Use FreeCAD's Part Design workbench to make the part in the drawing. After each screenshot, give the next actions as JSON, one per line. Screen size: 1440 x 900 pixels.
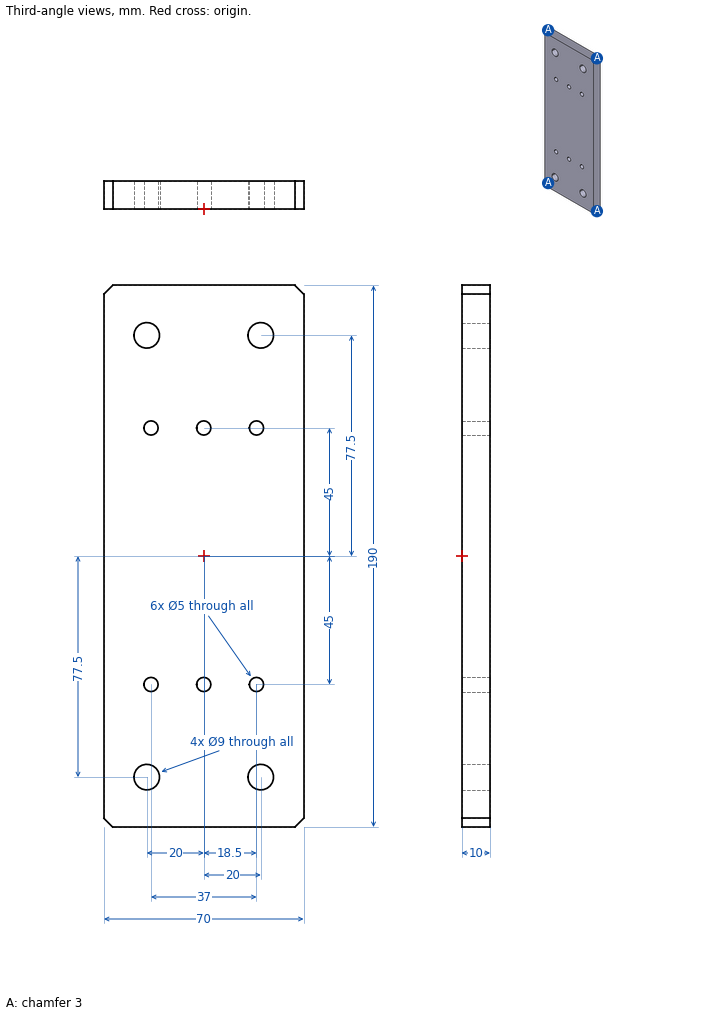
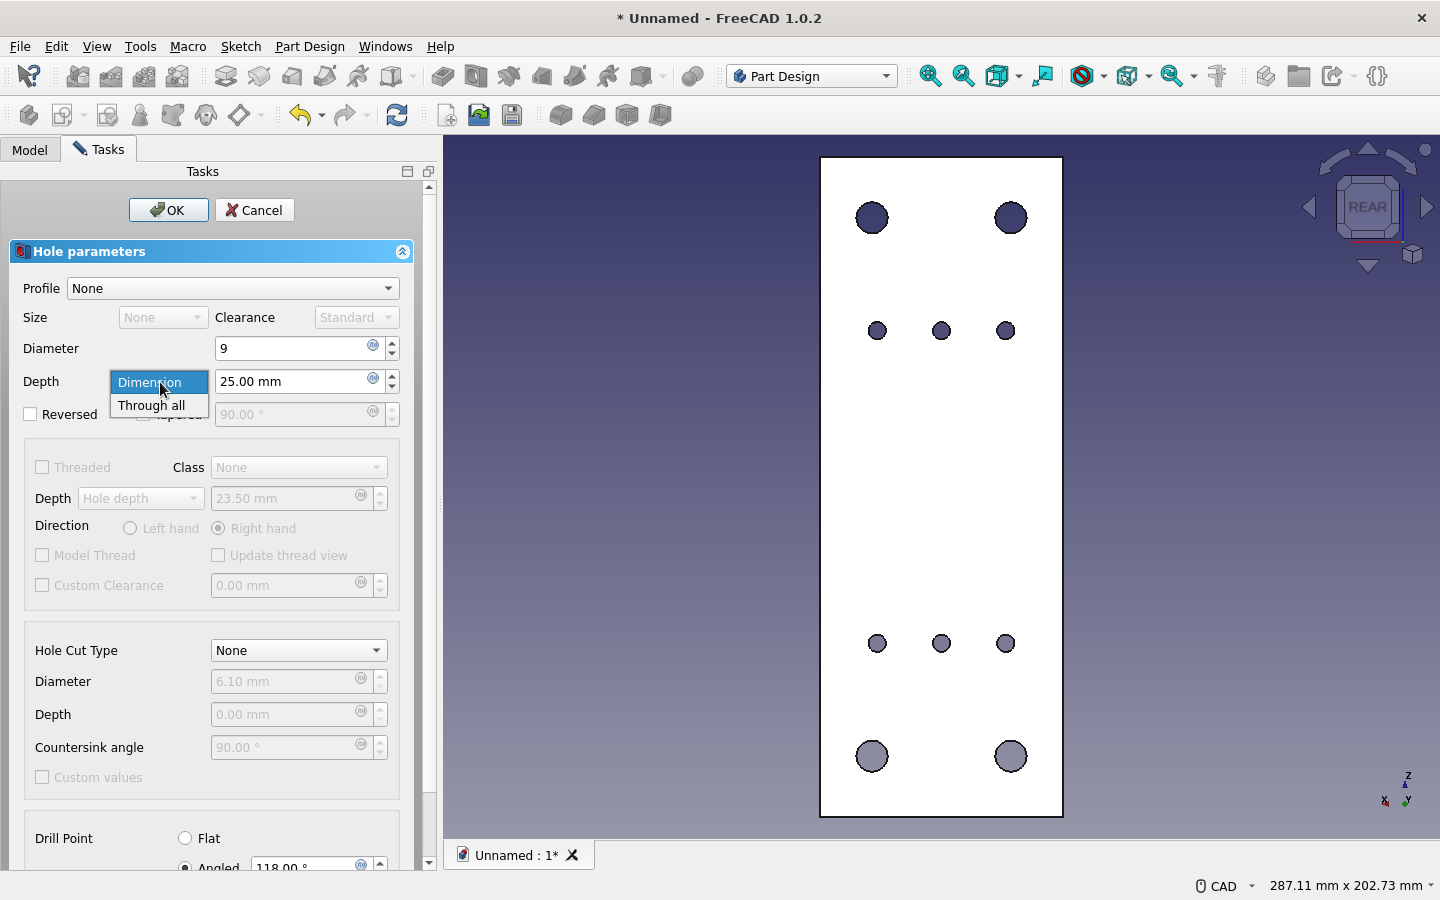
{"action": "left_click", "coordinate": [158, 406]}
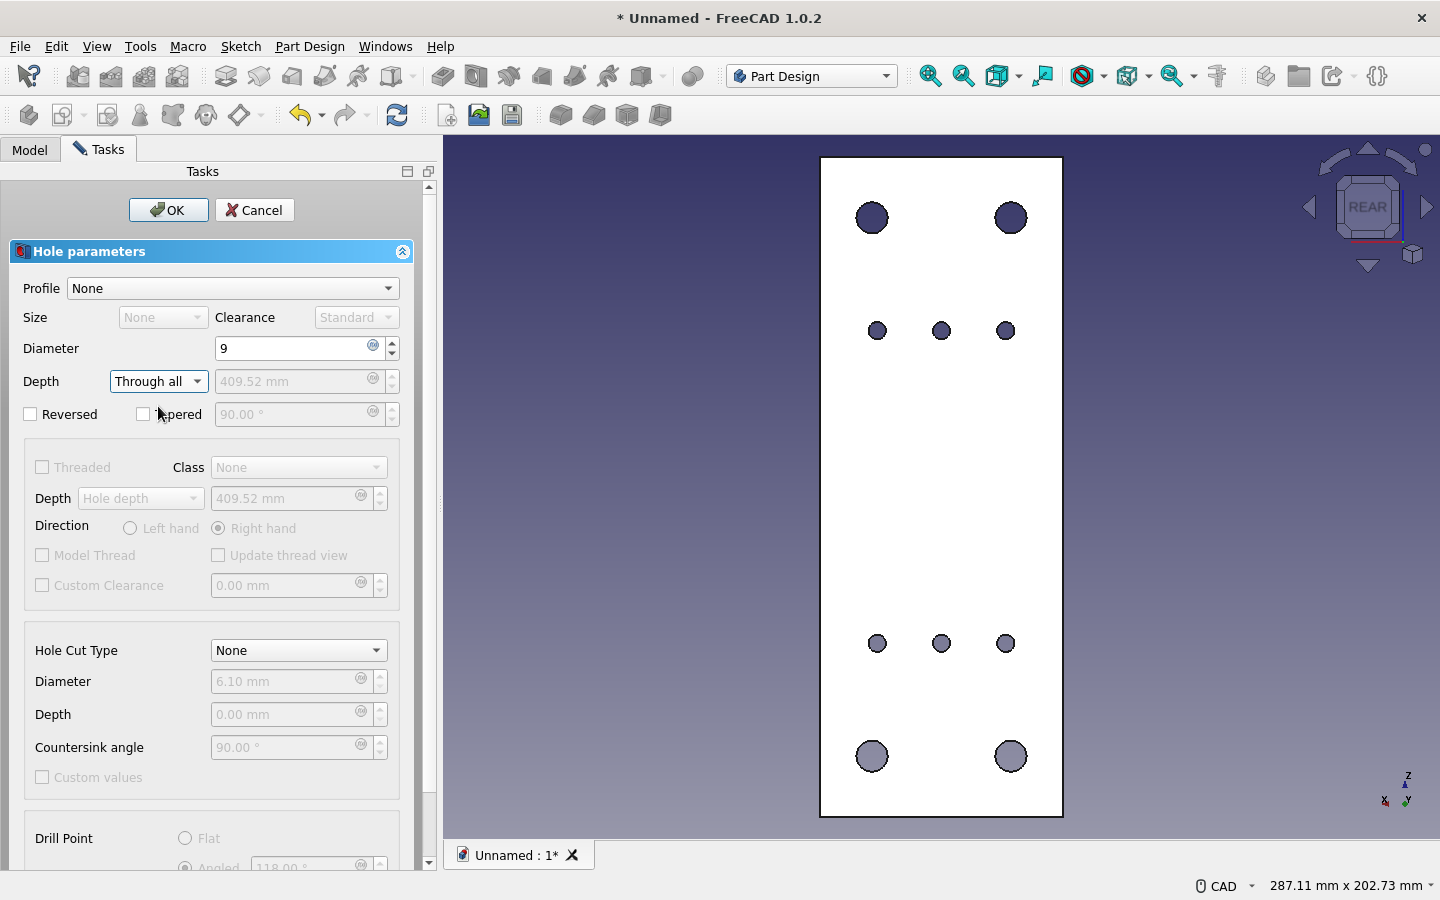
{"action": "left_click", "coordinate": [169, 210]}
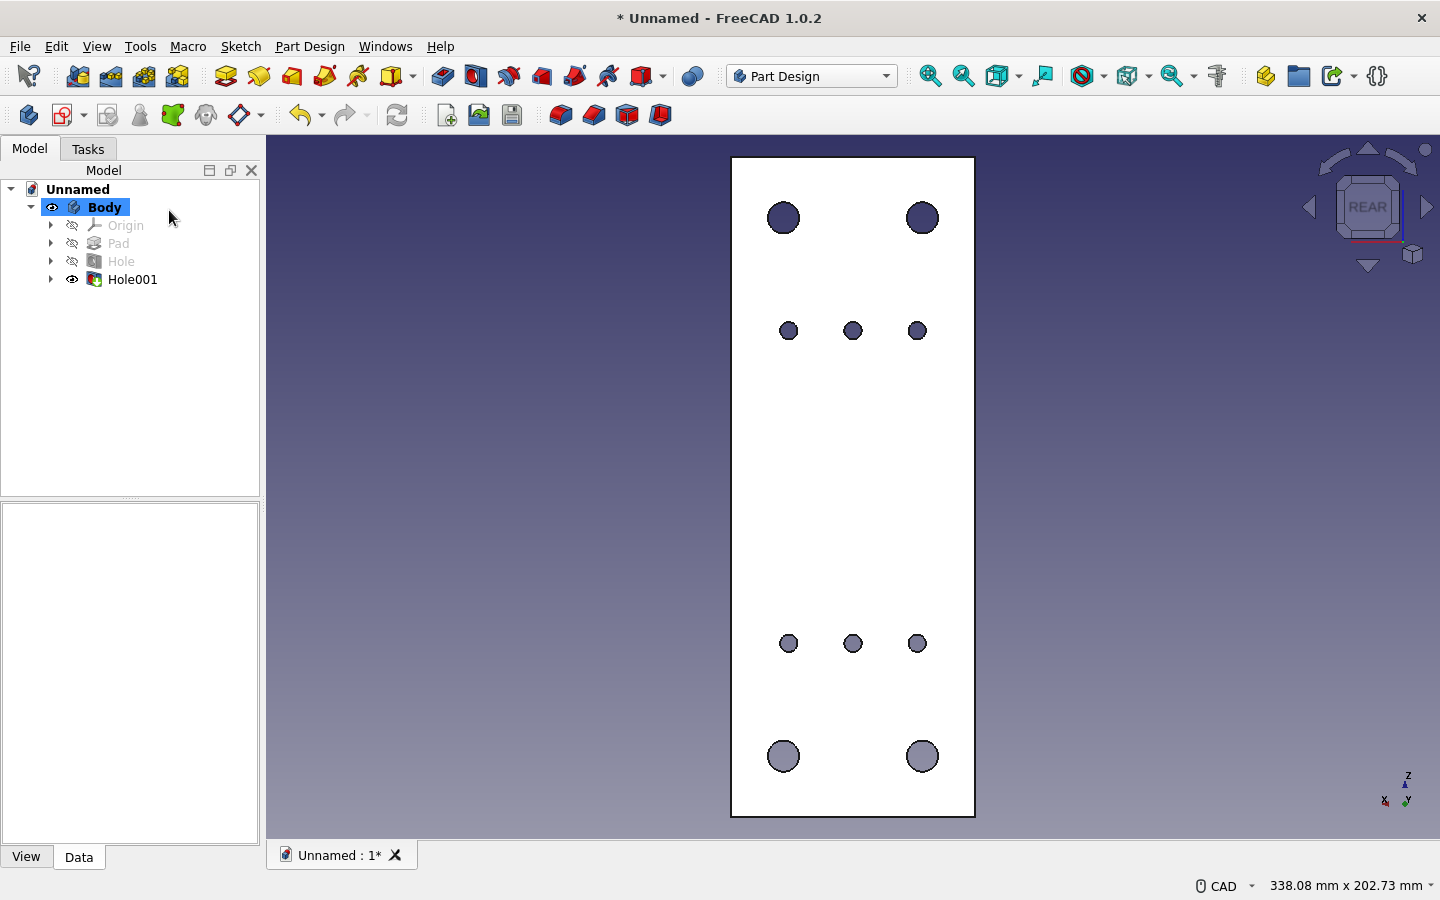
{"action": "key", "text": "0"}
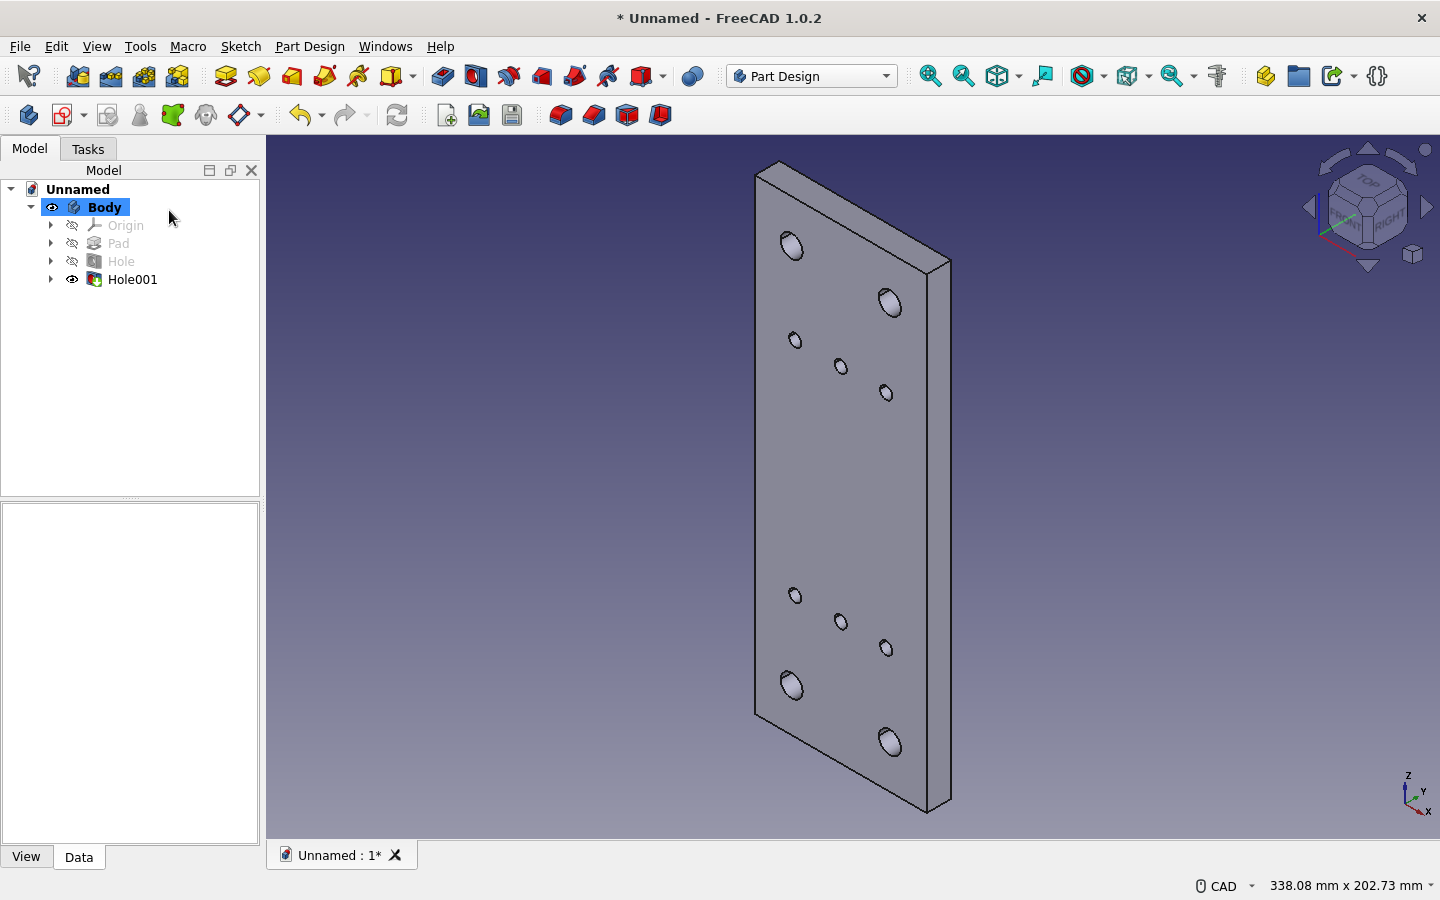
{"action": "left_click", "coordinate": [939, 266]}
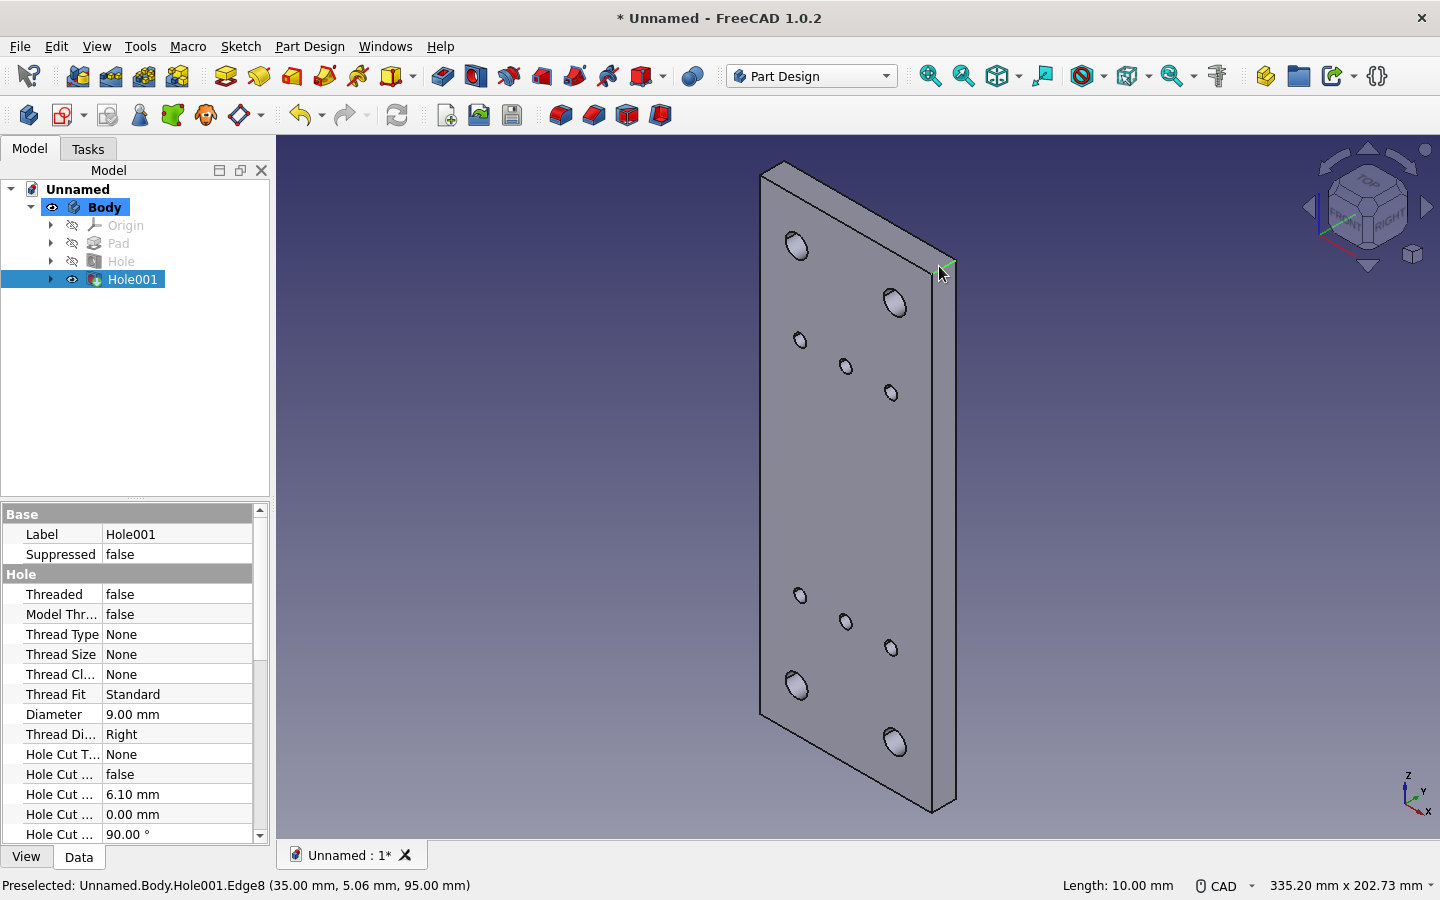
{"action": "key", "text": "2"}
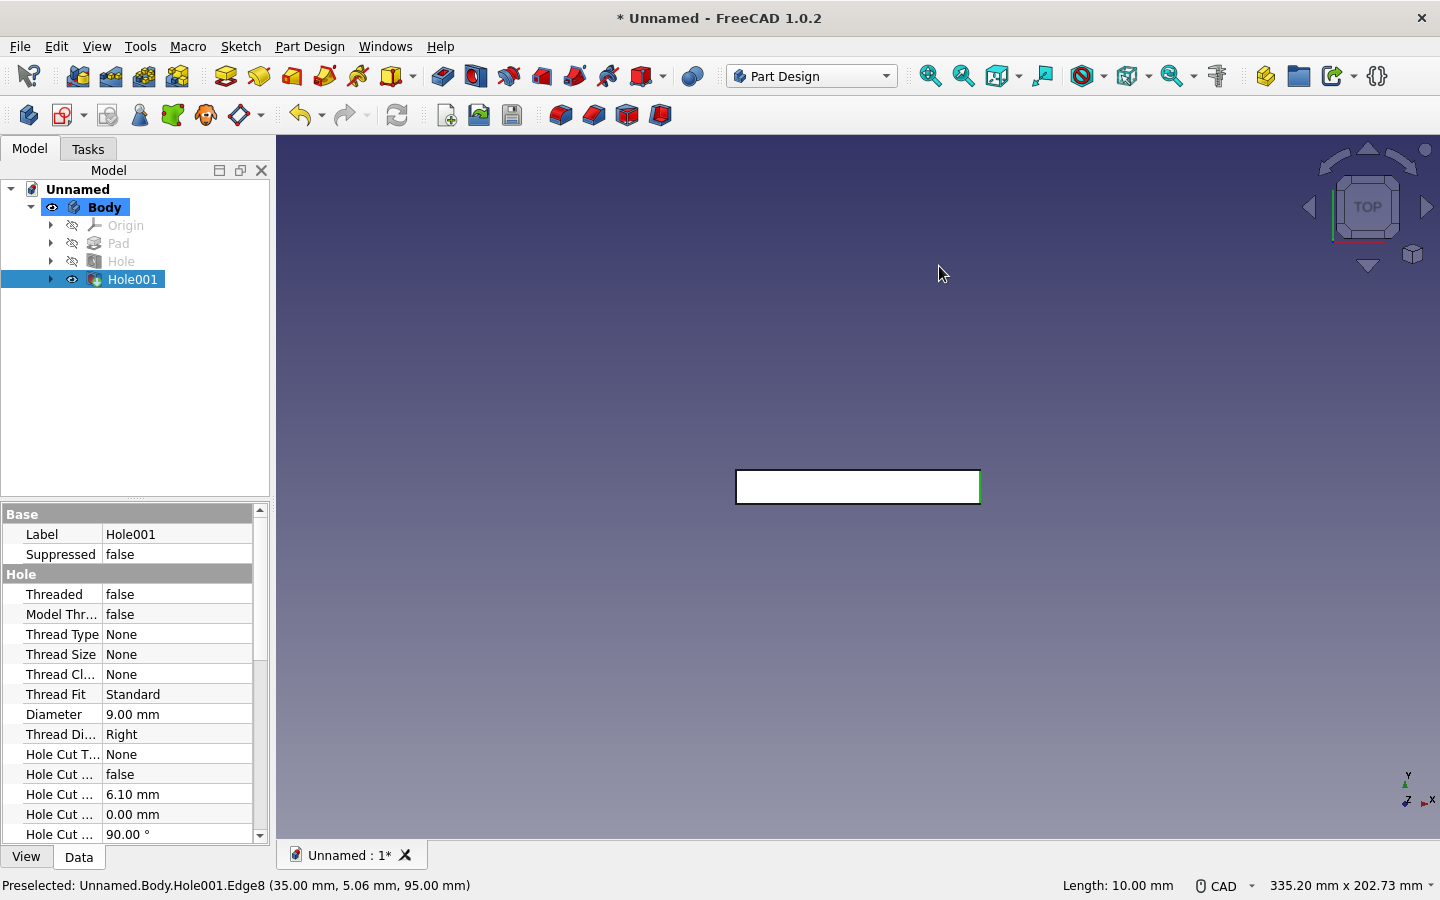
{"action": "key", "text": "v f"}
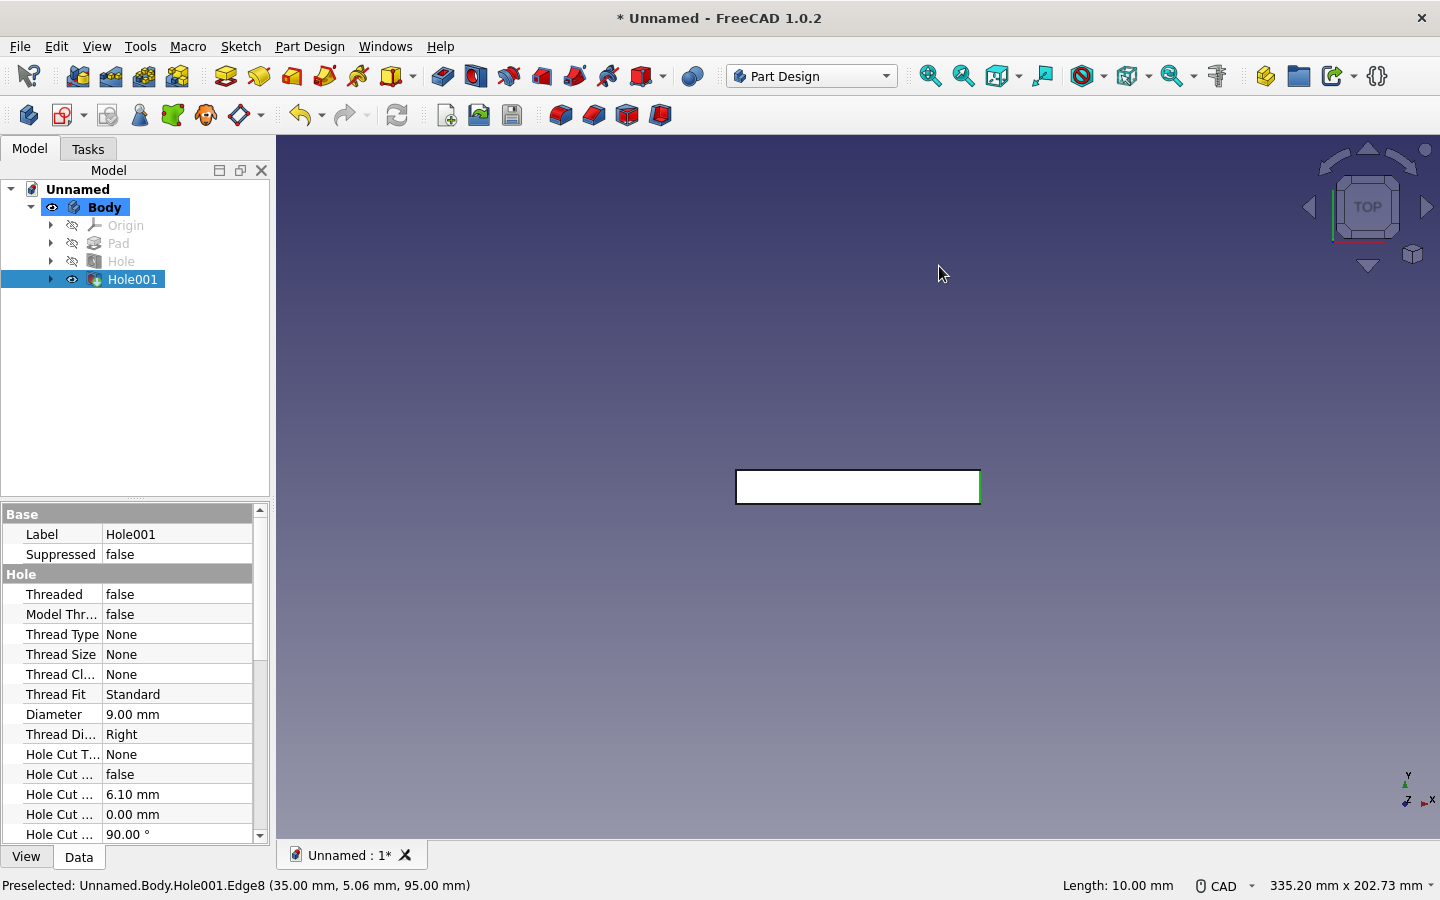
{"action": "left_click", "coordinate": [736, 486], "text": "ctrl"}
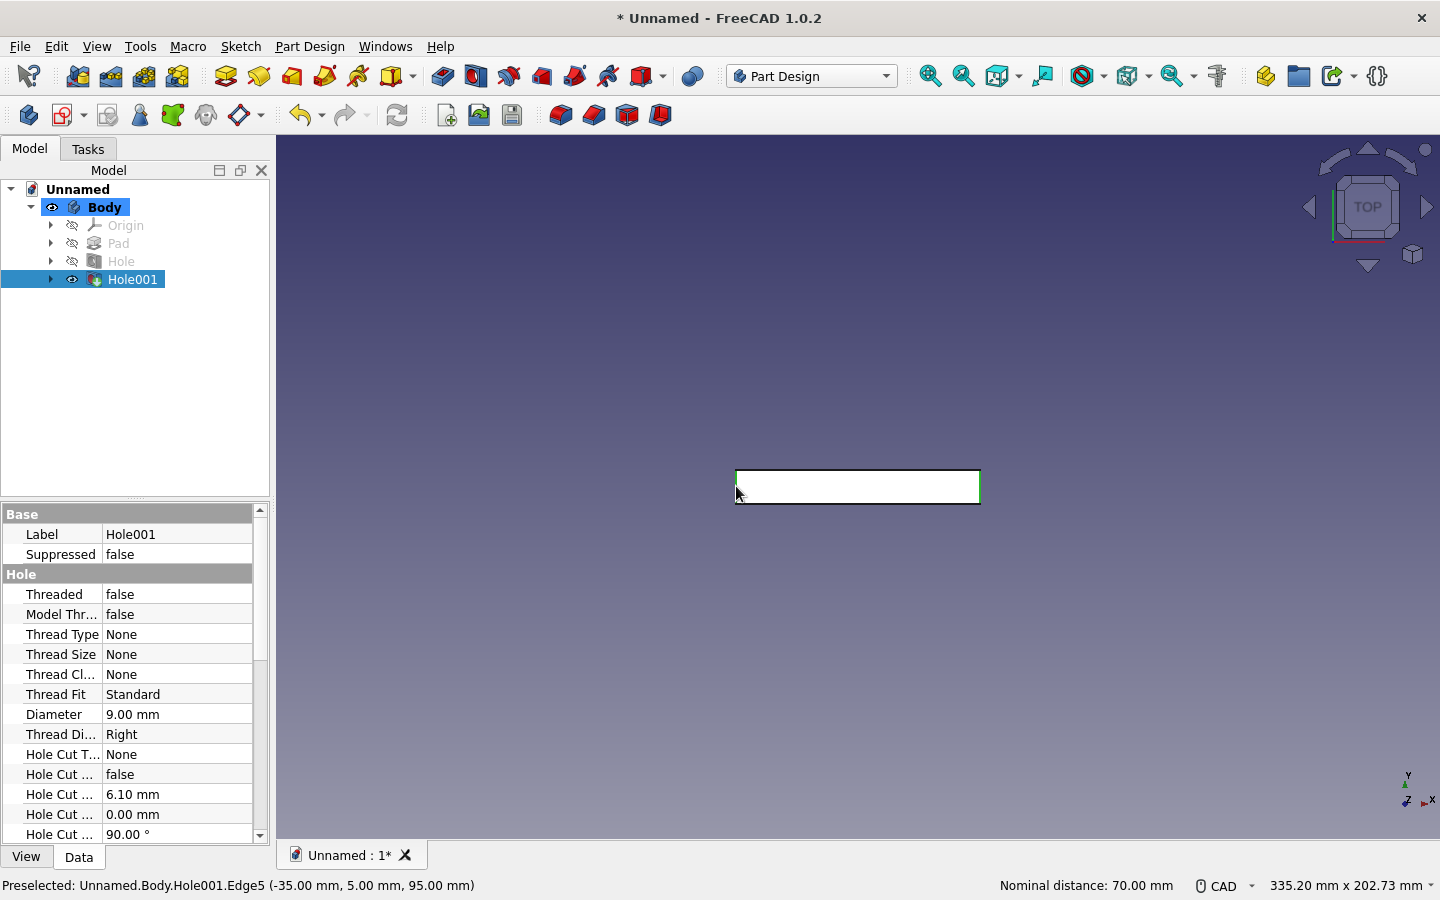
{"action": "key", "text": "1"}